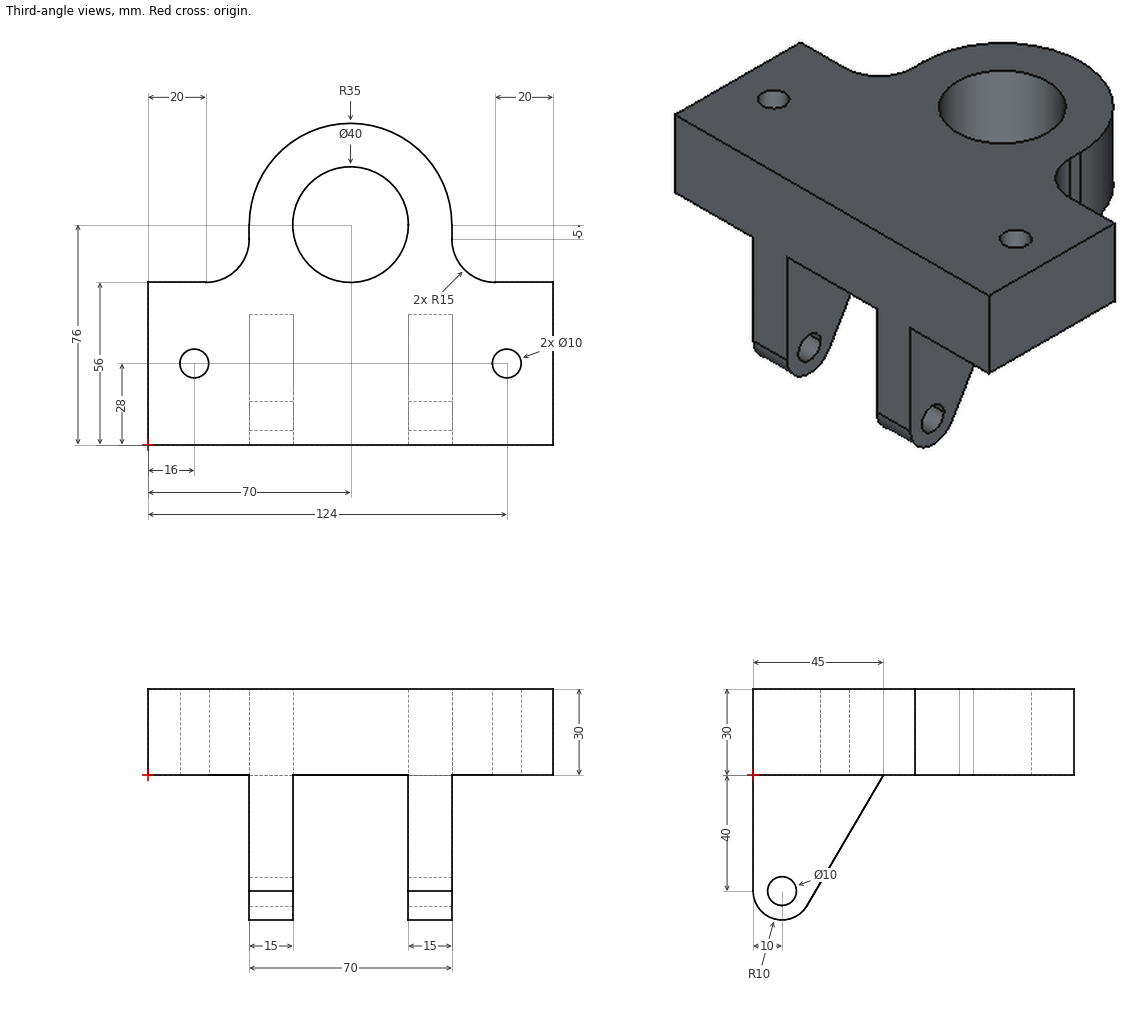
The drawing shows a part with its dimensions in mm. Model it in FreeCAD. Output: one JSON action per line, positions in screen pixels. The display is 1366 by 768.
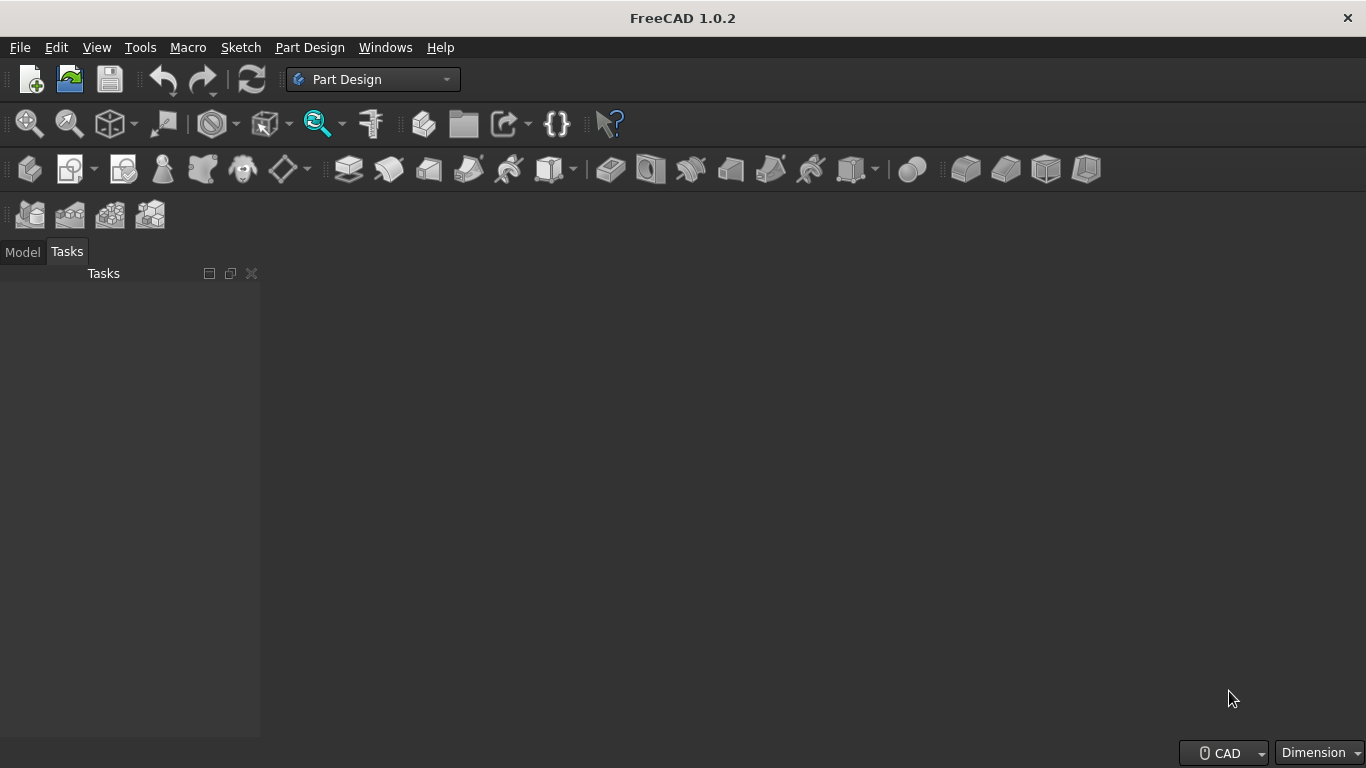
{"action": "left_click", "coordinate": [30, 80]}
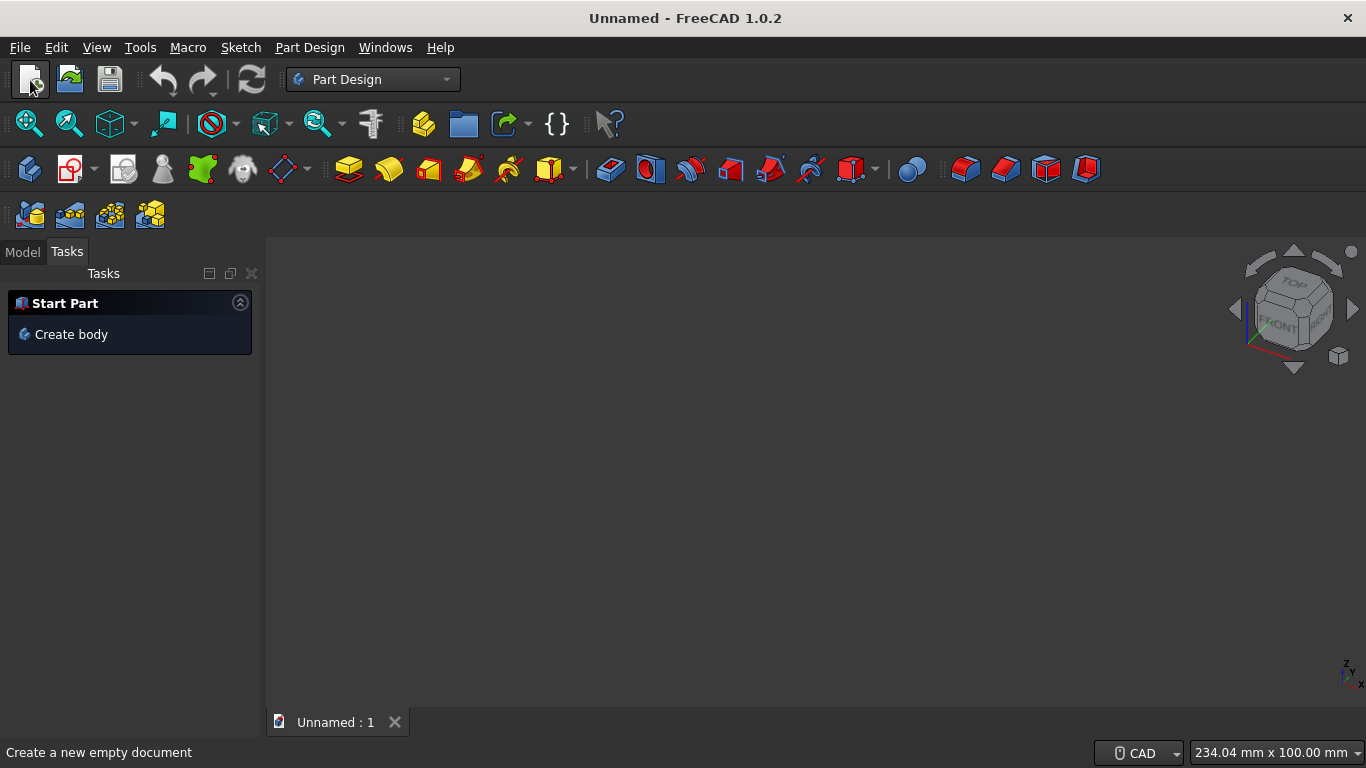
{"action": "left_click", "coordinate": [70, 170]}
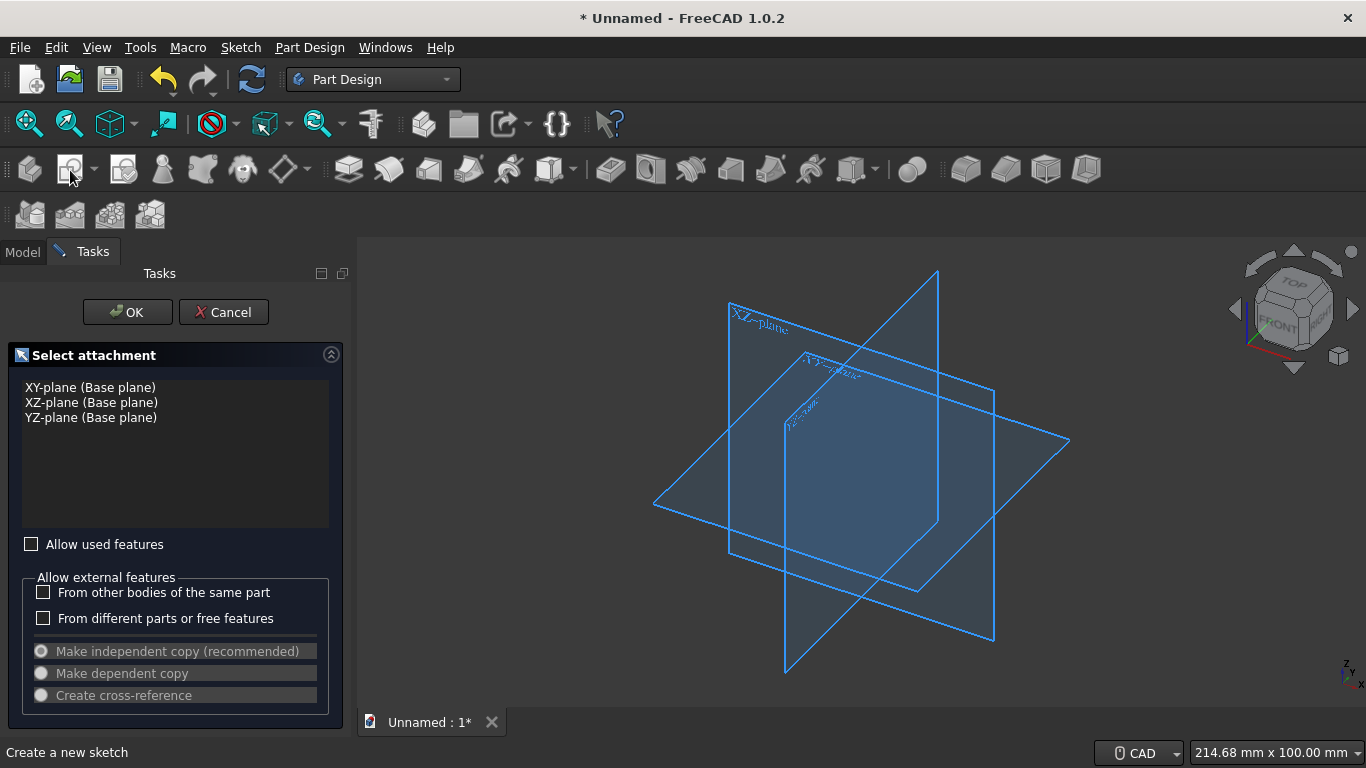
{"action": "left_click", "coordinate": [82, 388]}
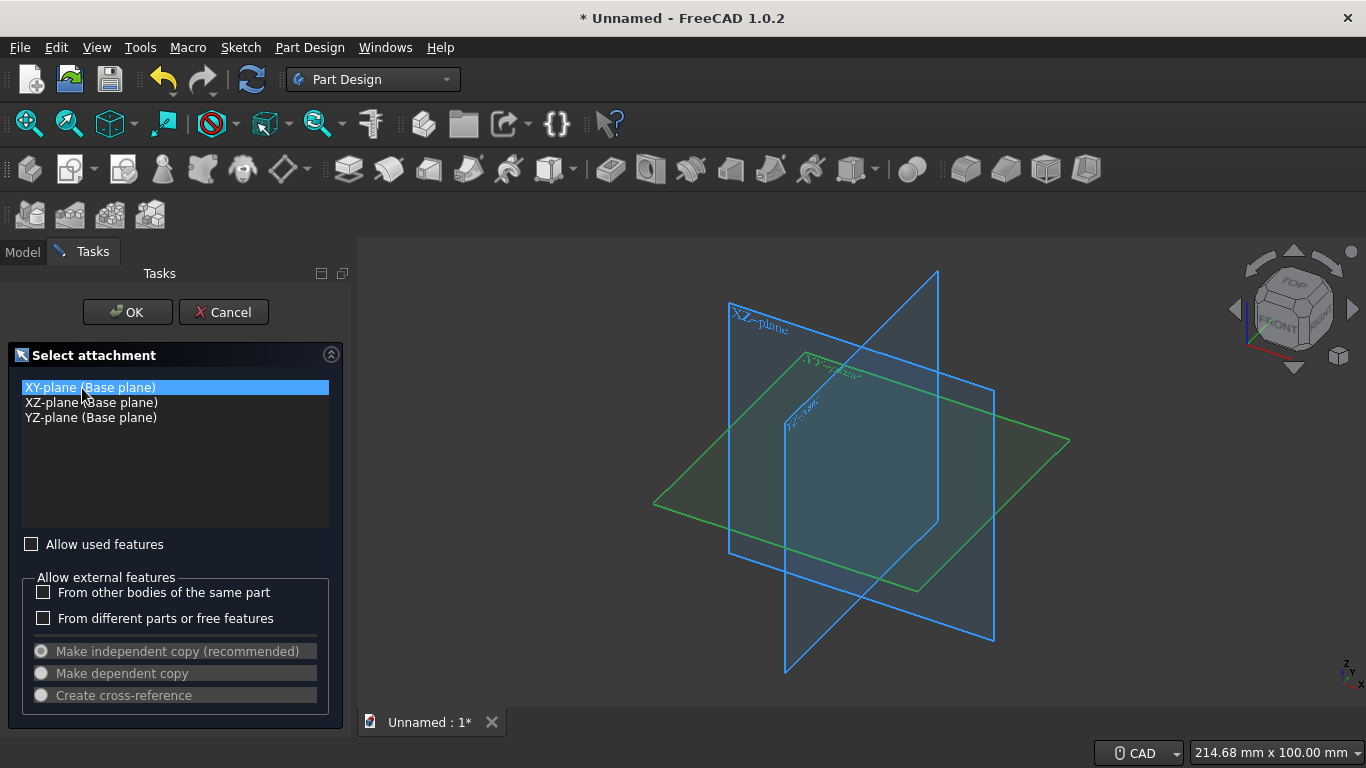
{"action": "left_click", "coordinate": [128, 312]}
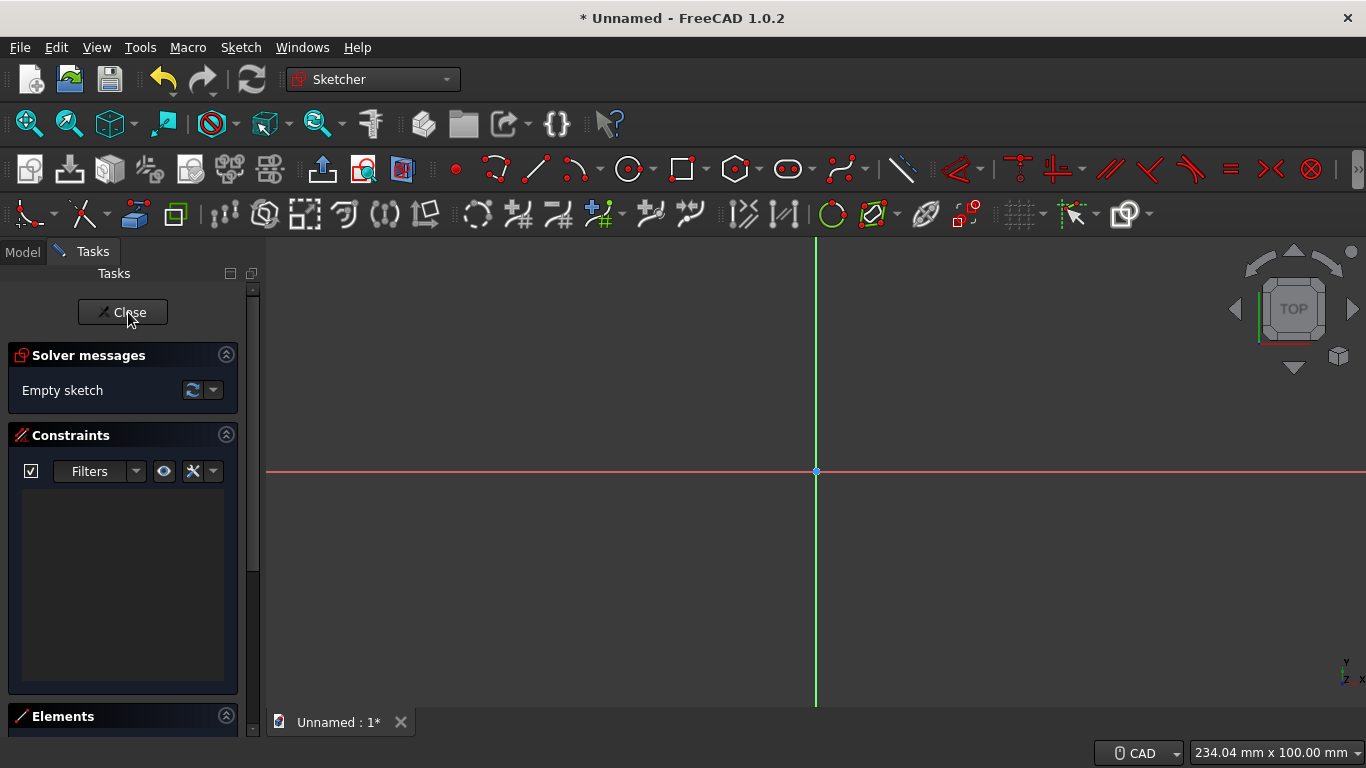
{"action": "scroll", "coordinate": [423, 679], "scroll_direction": "down", "scroll_amount": 4}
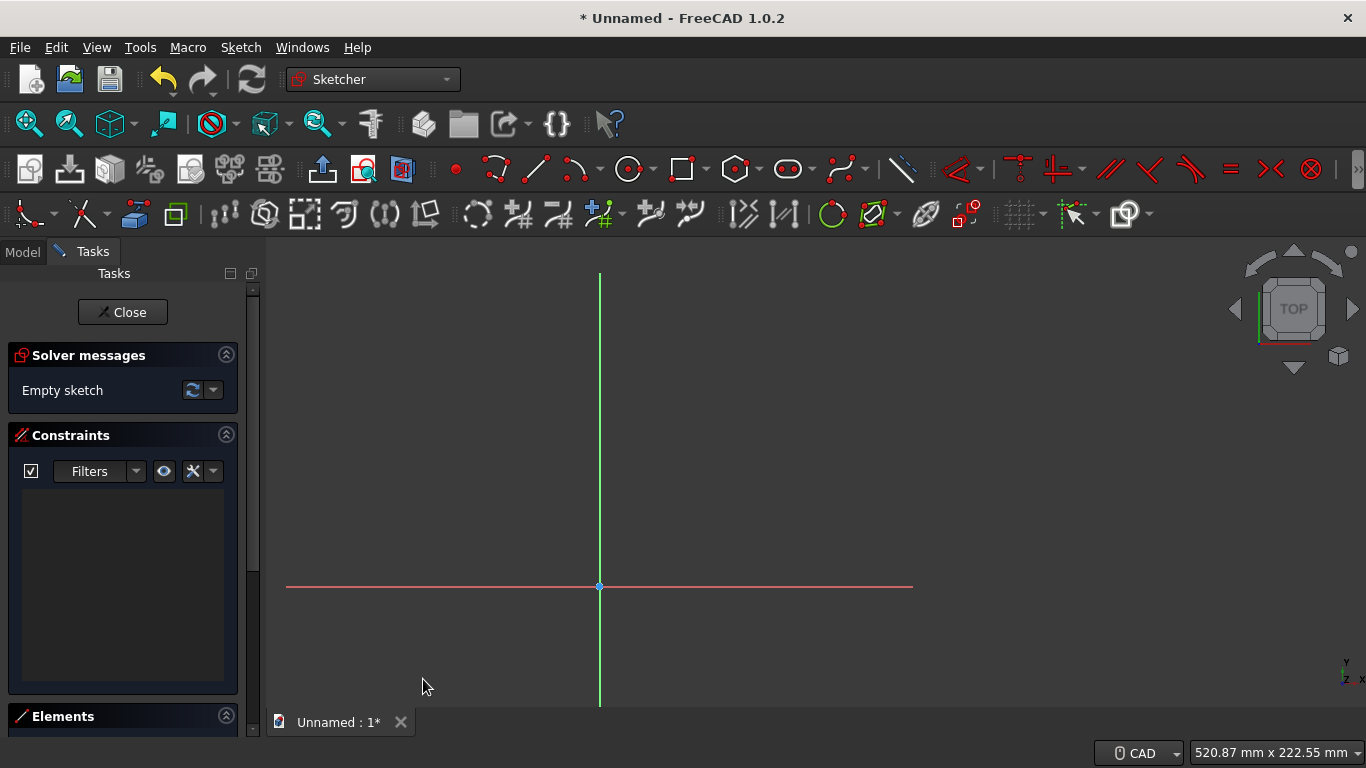
{"action": "left_click", "coordinate": [536, 170]}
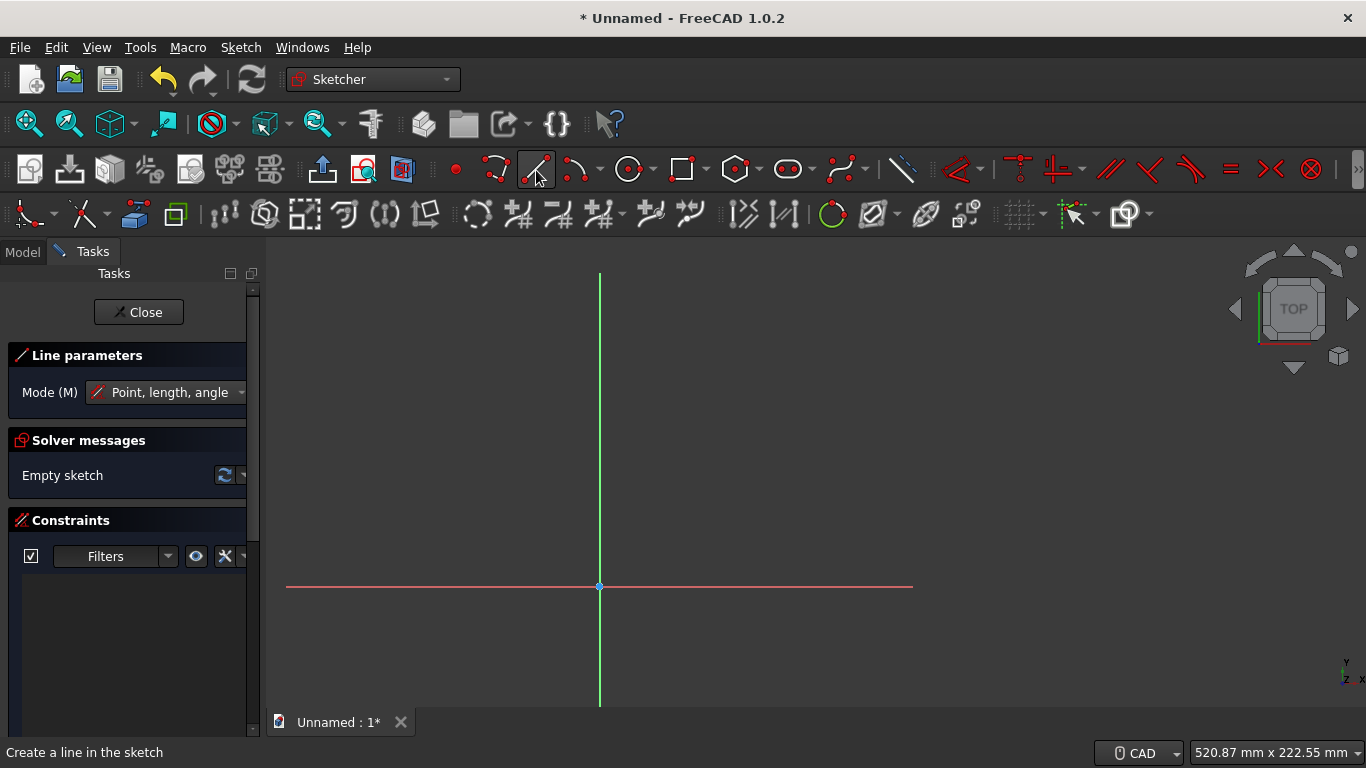
{"action": "left_click", "coordinate": [821, 437]}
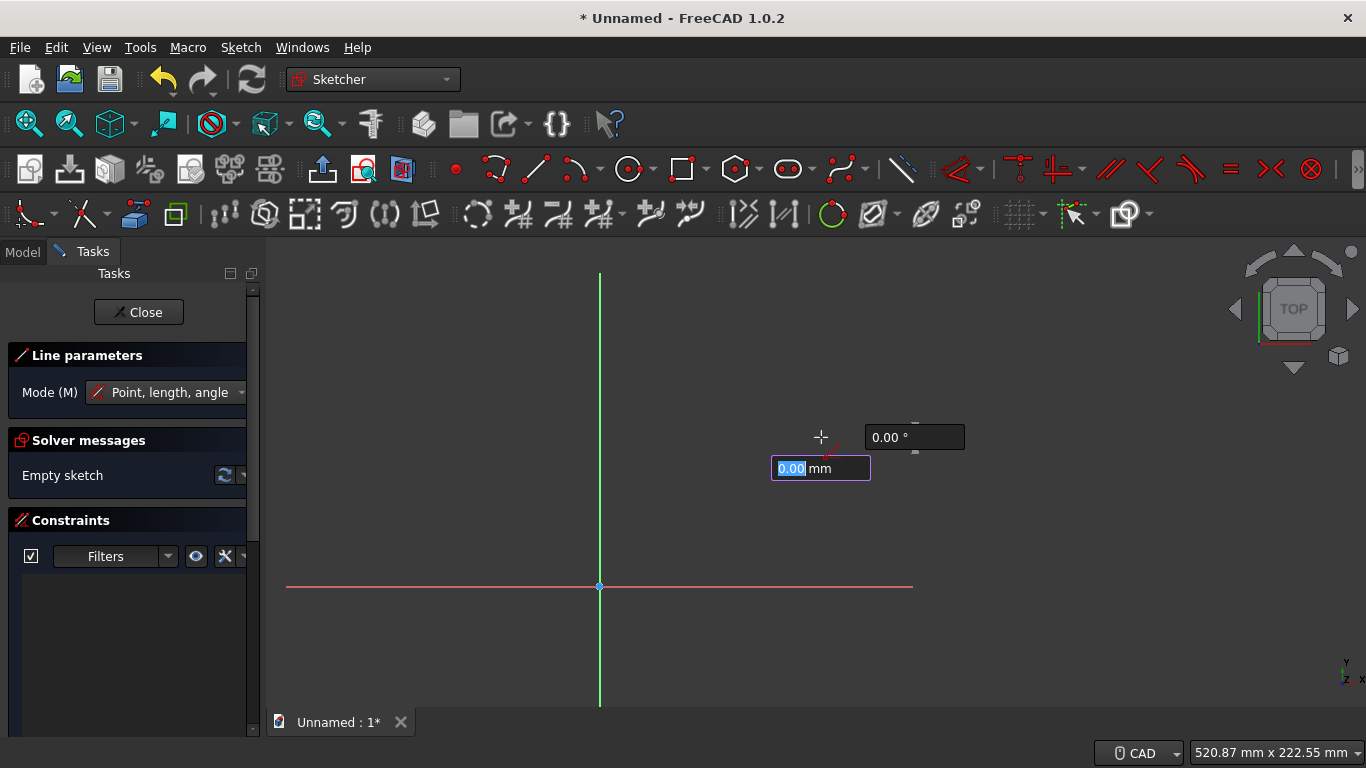
{"action": "scroll", "coordinate": [821, 426], "scroll_direction": "up", "scroll_amount": 3}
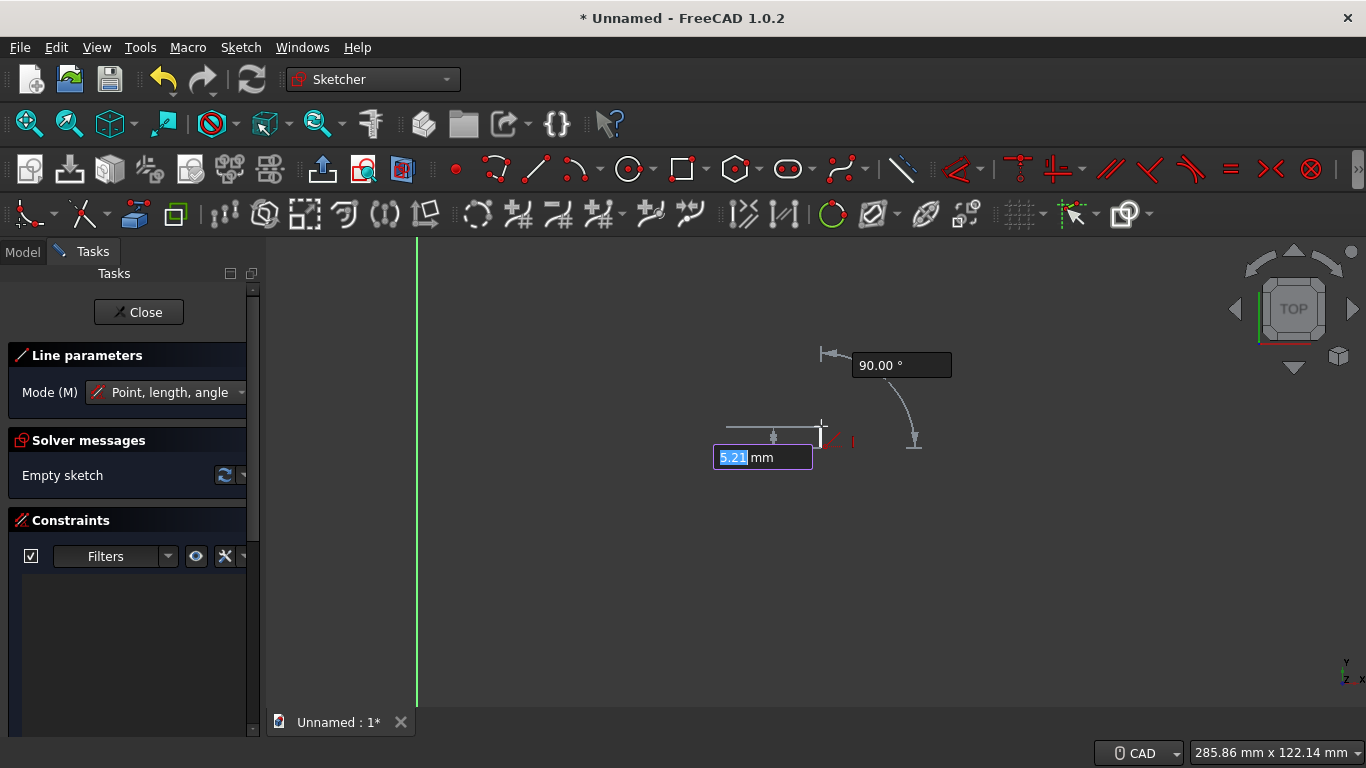
{"action": "left_click", "coordinate": [821, 426]}